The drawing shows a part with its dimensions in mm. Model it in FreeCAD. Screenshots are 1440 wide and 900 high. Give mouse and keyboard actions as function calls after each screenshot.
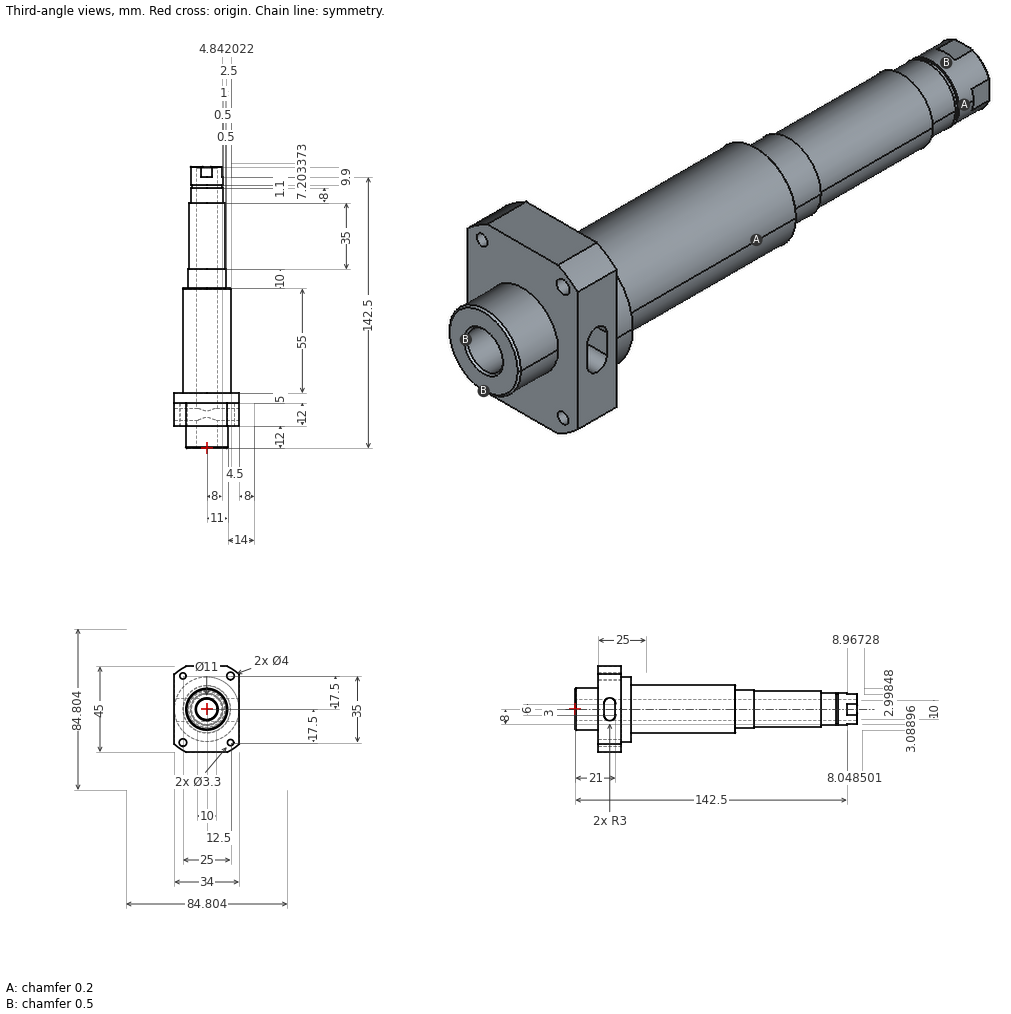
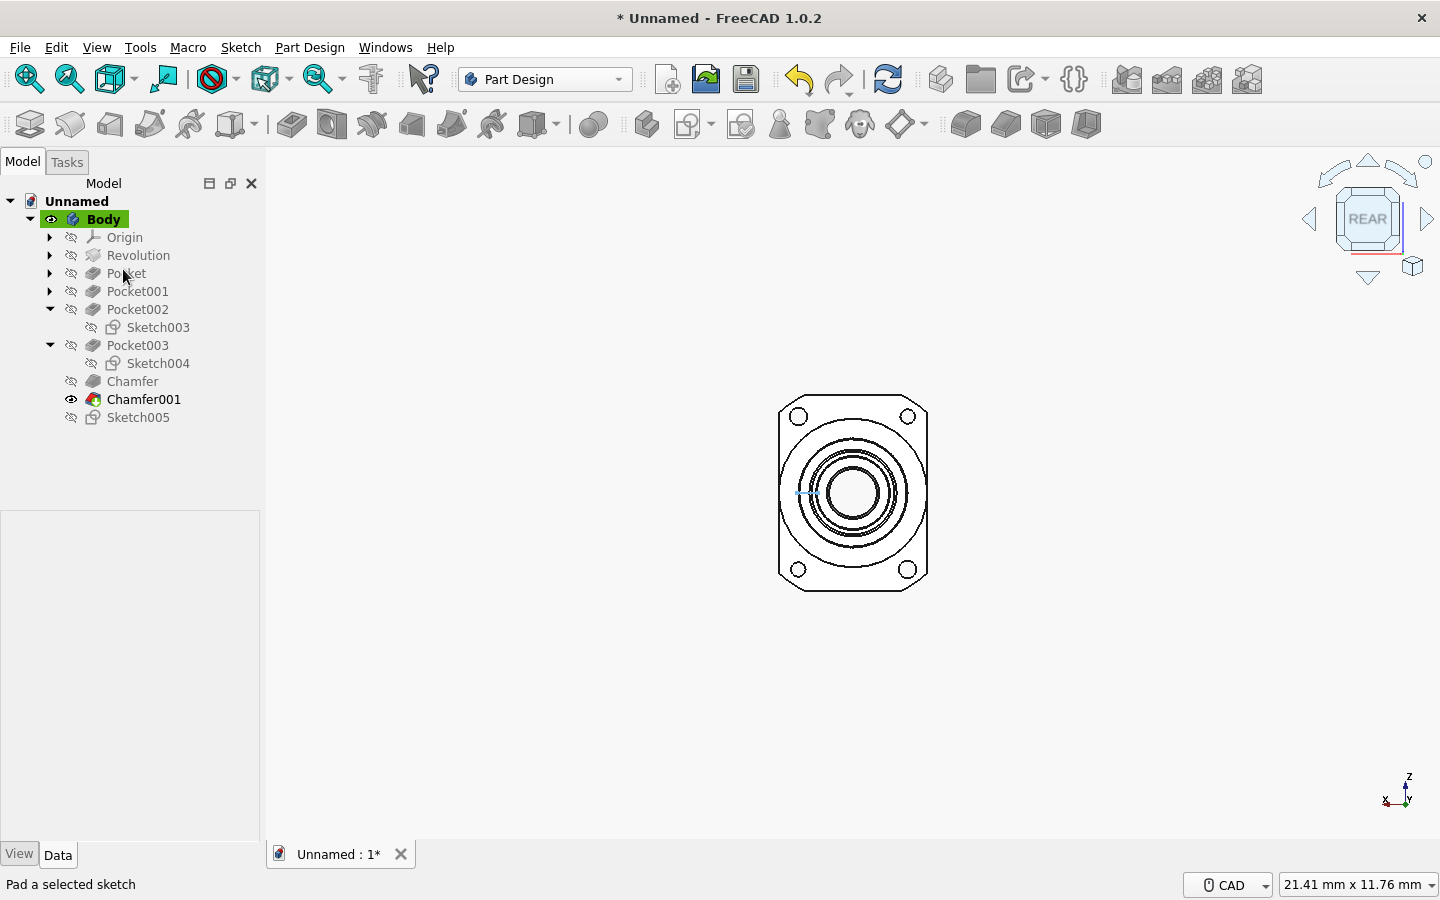
click(292, 124)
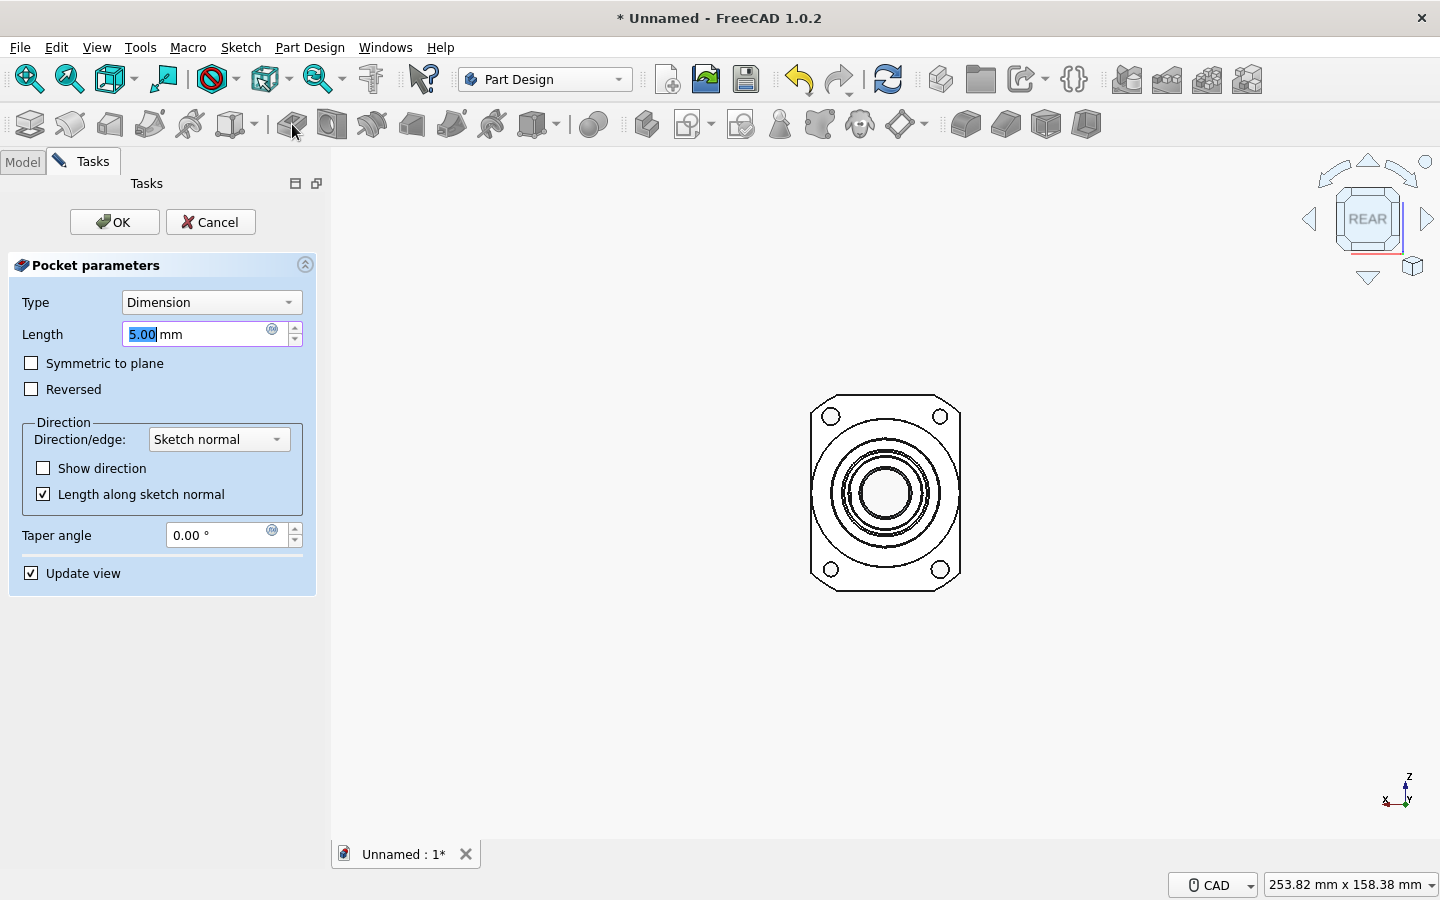
text(10)
key(Tab)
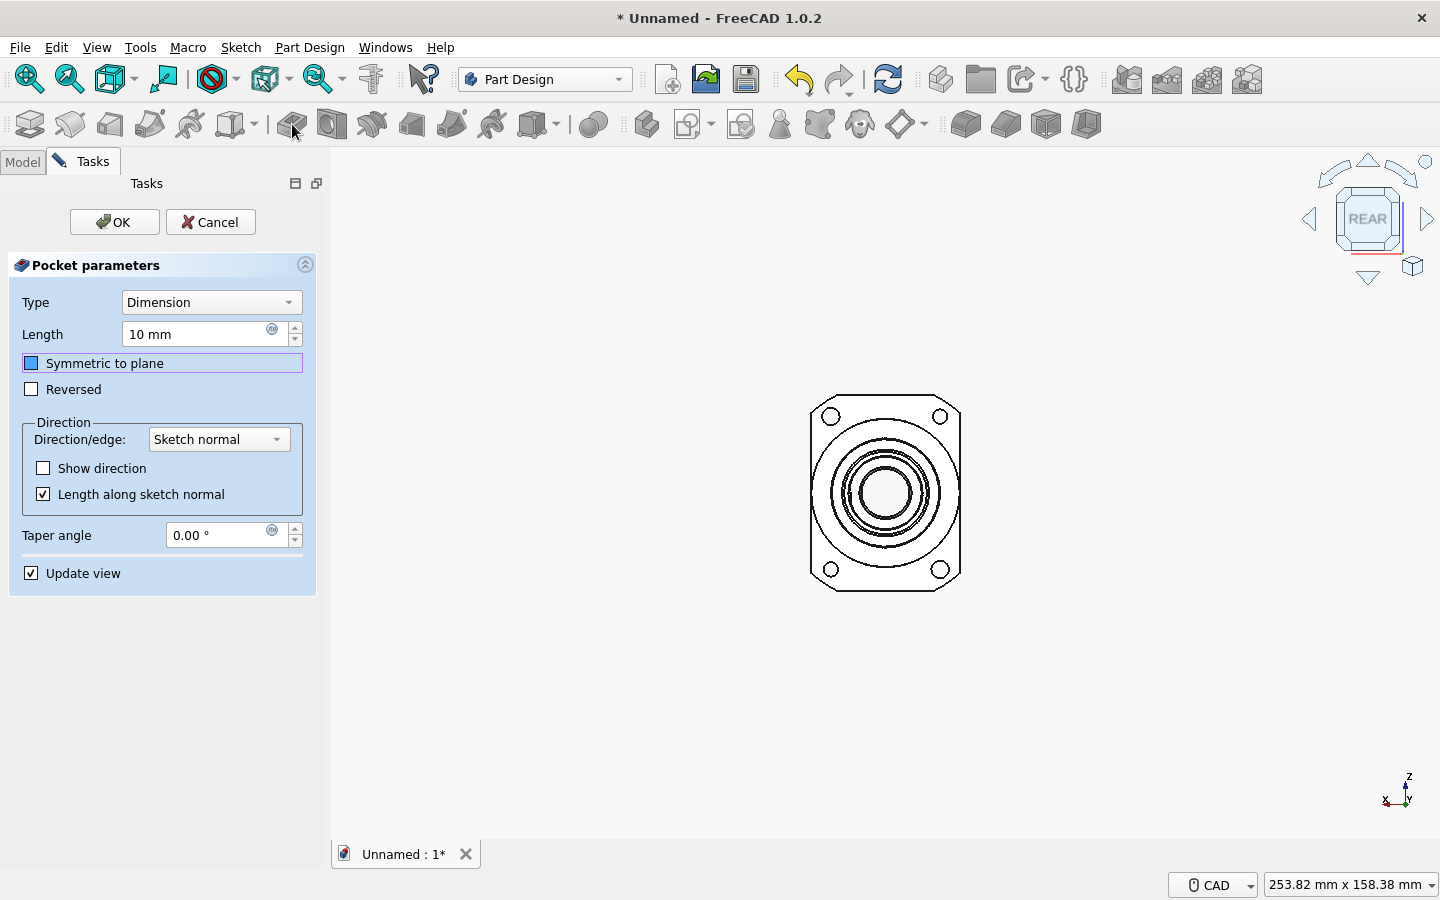
click(30, 363)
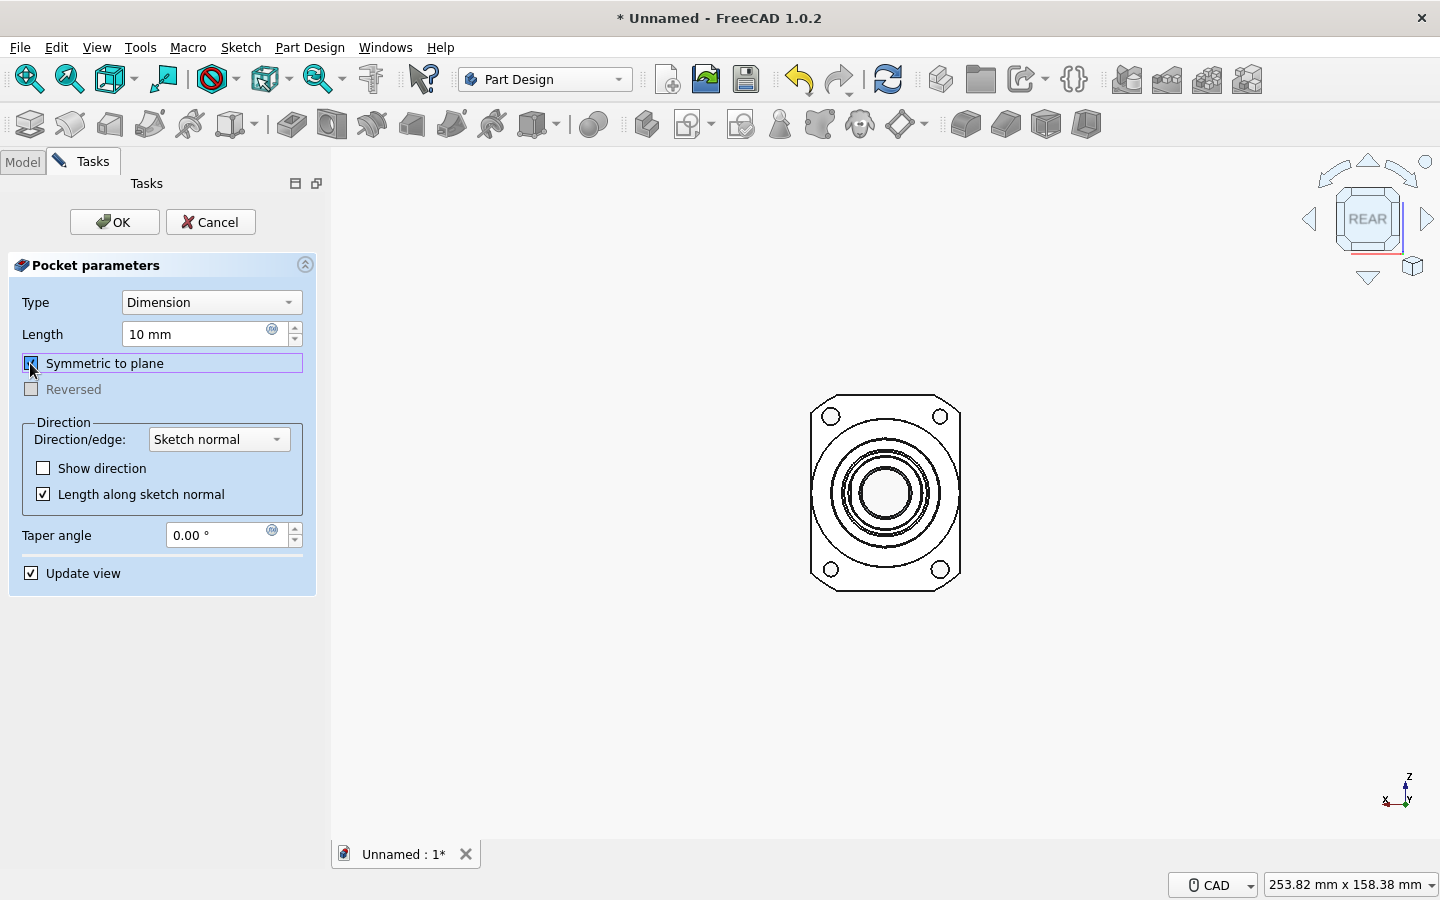
click(115, 222)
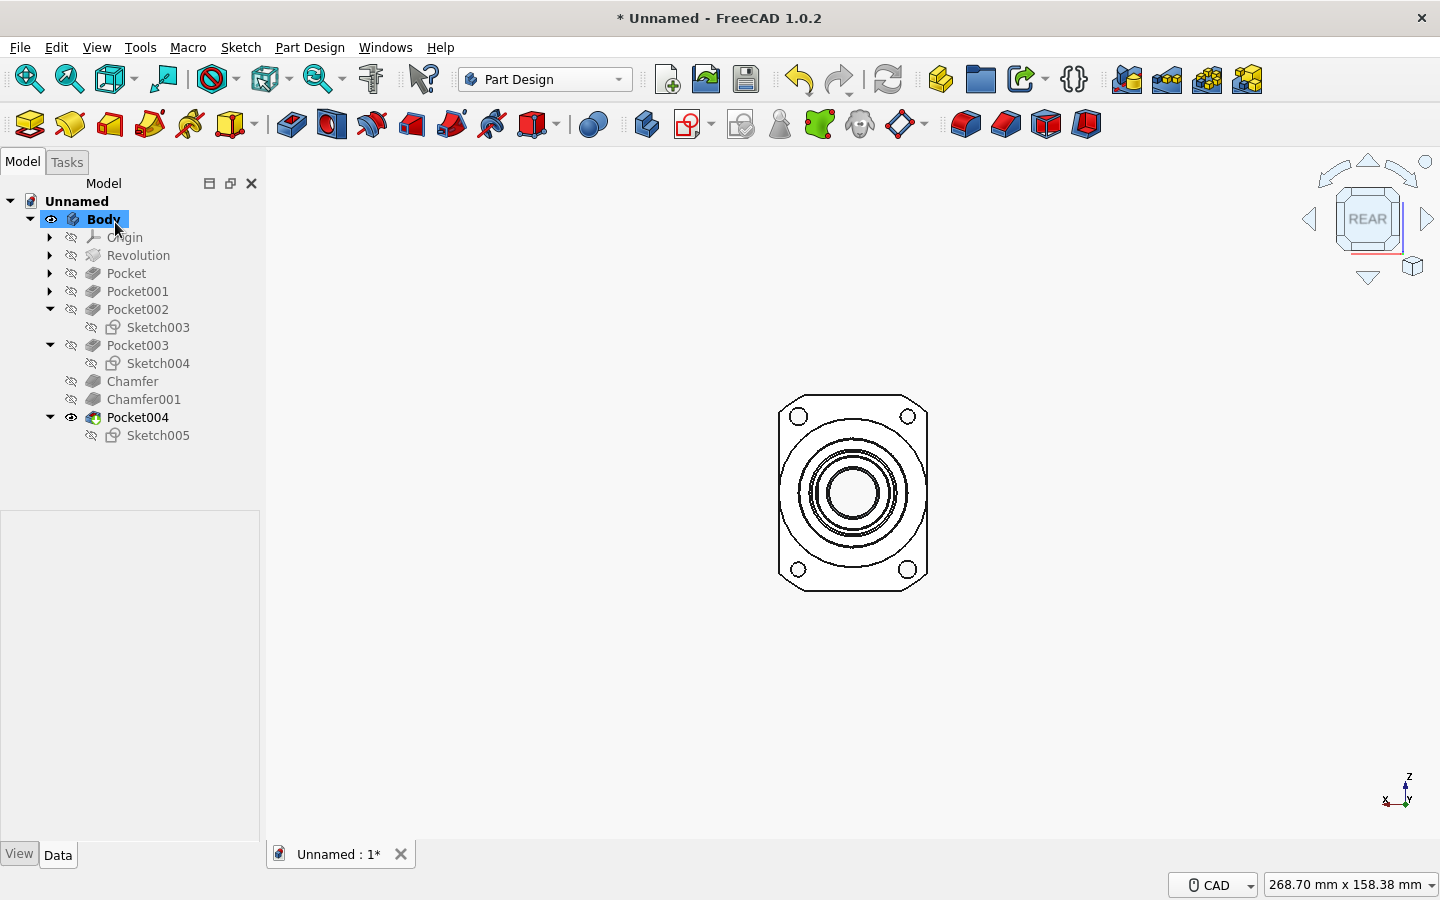
click(30, 80)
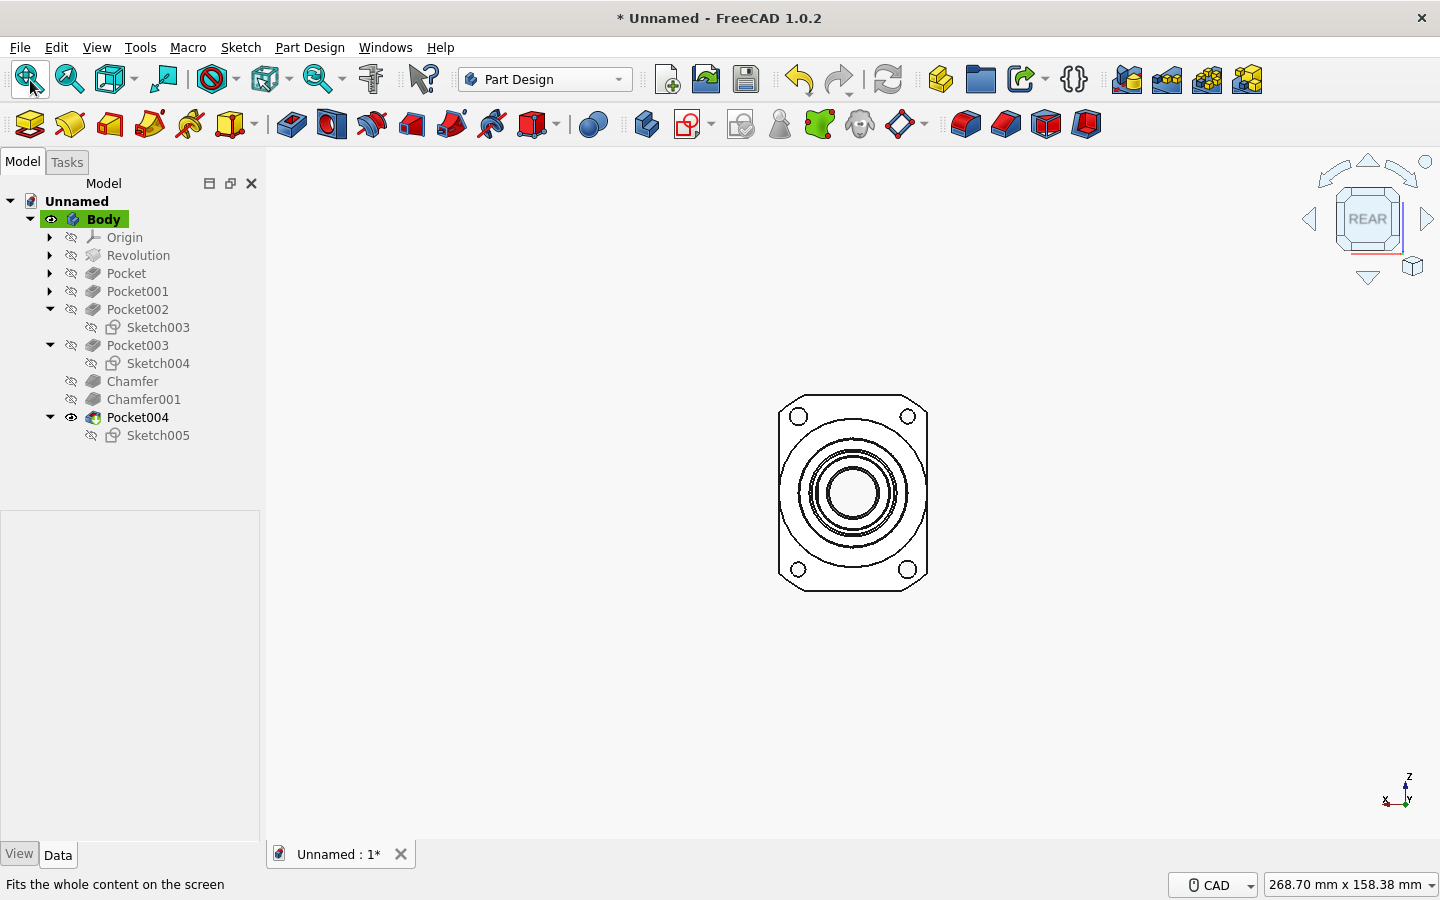
key(6)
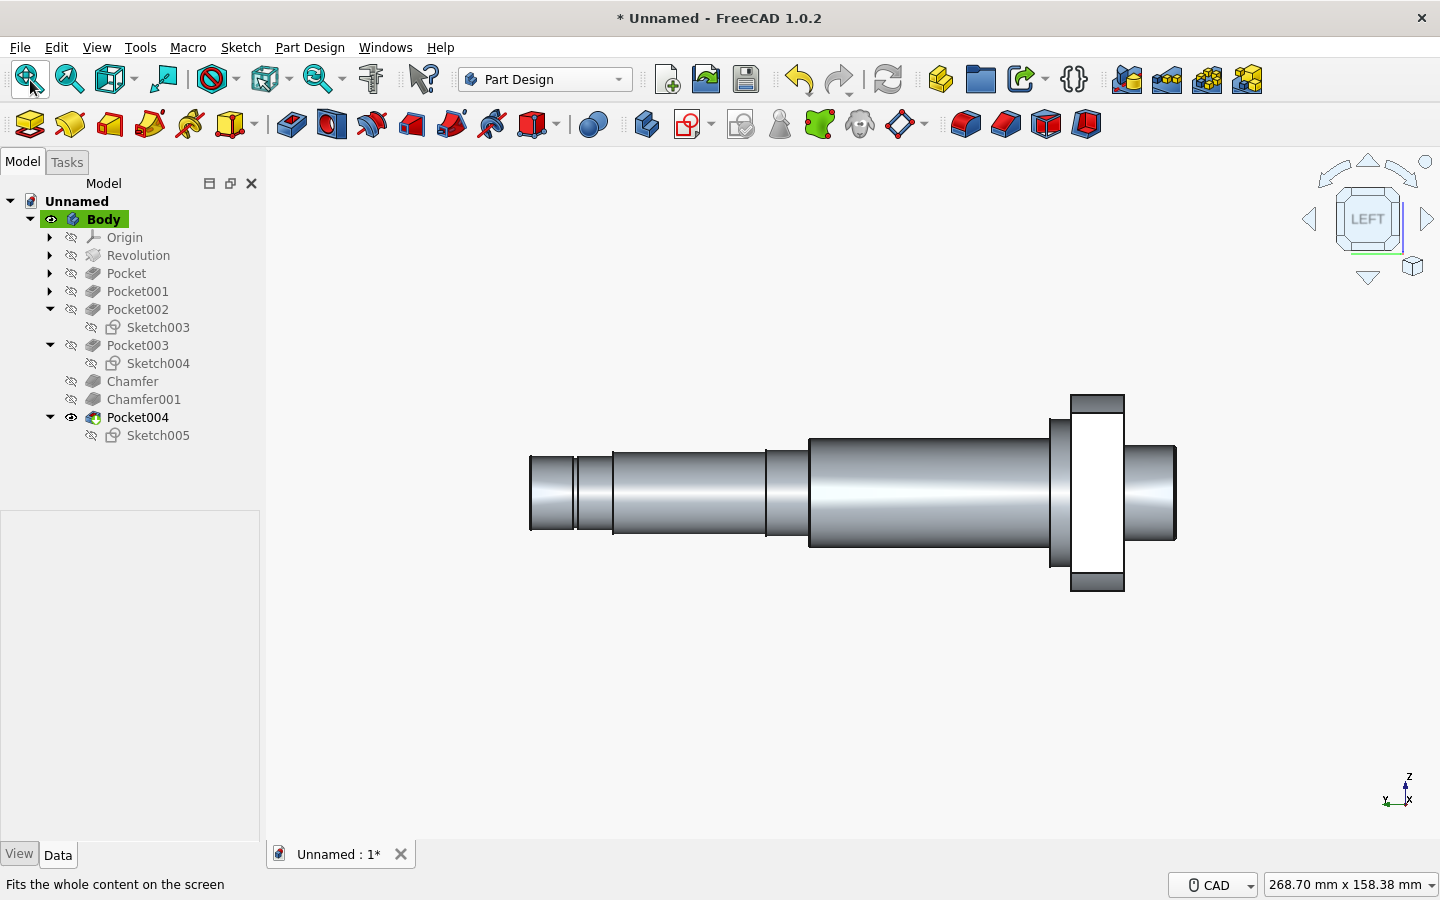
click(1098, 446)